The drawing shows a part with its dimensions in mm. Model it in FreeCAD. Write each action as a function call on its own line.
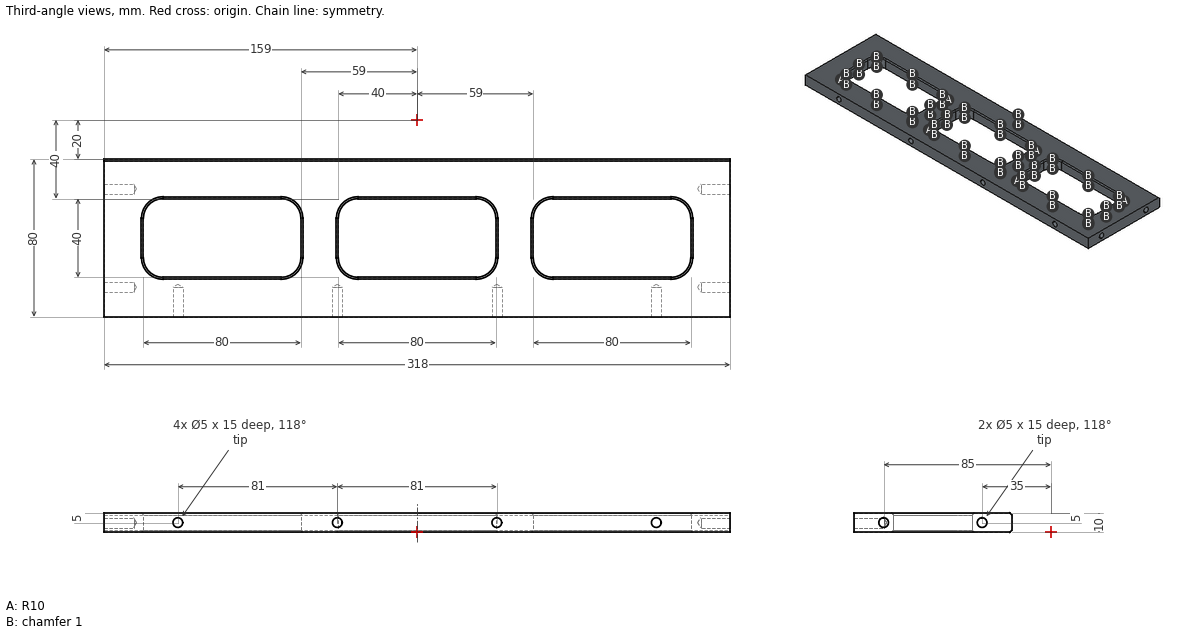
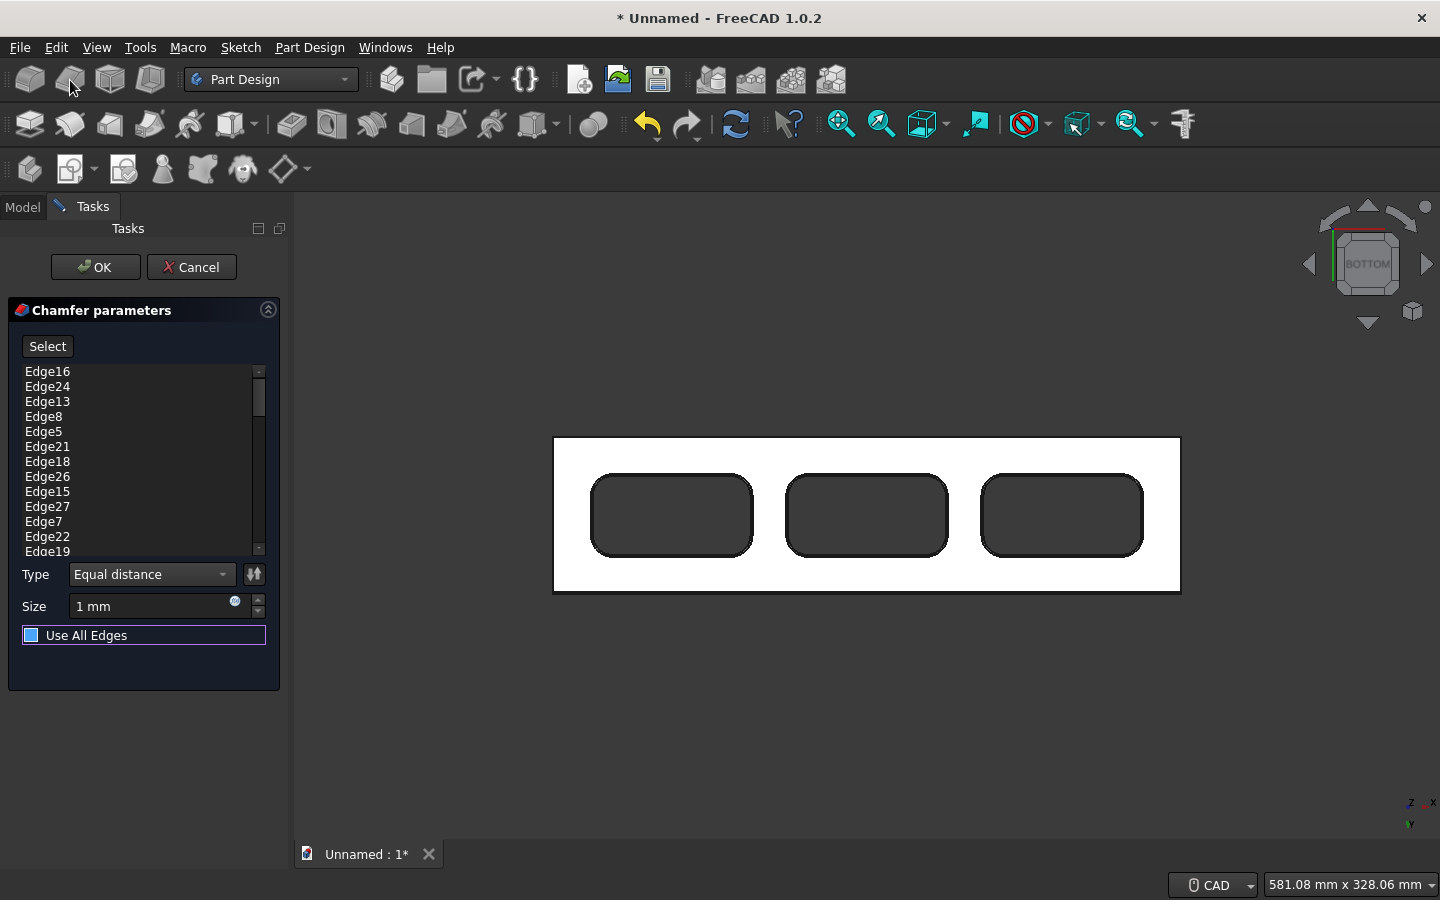
click(96, 267)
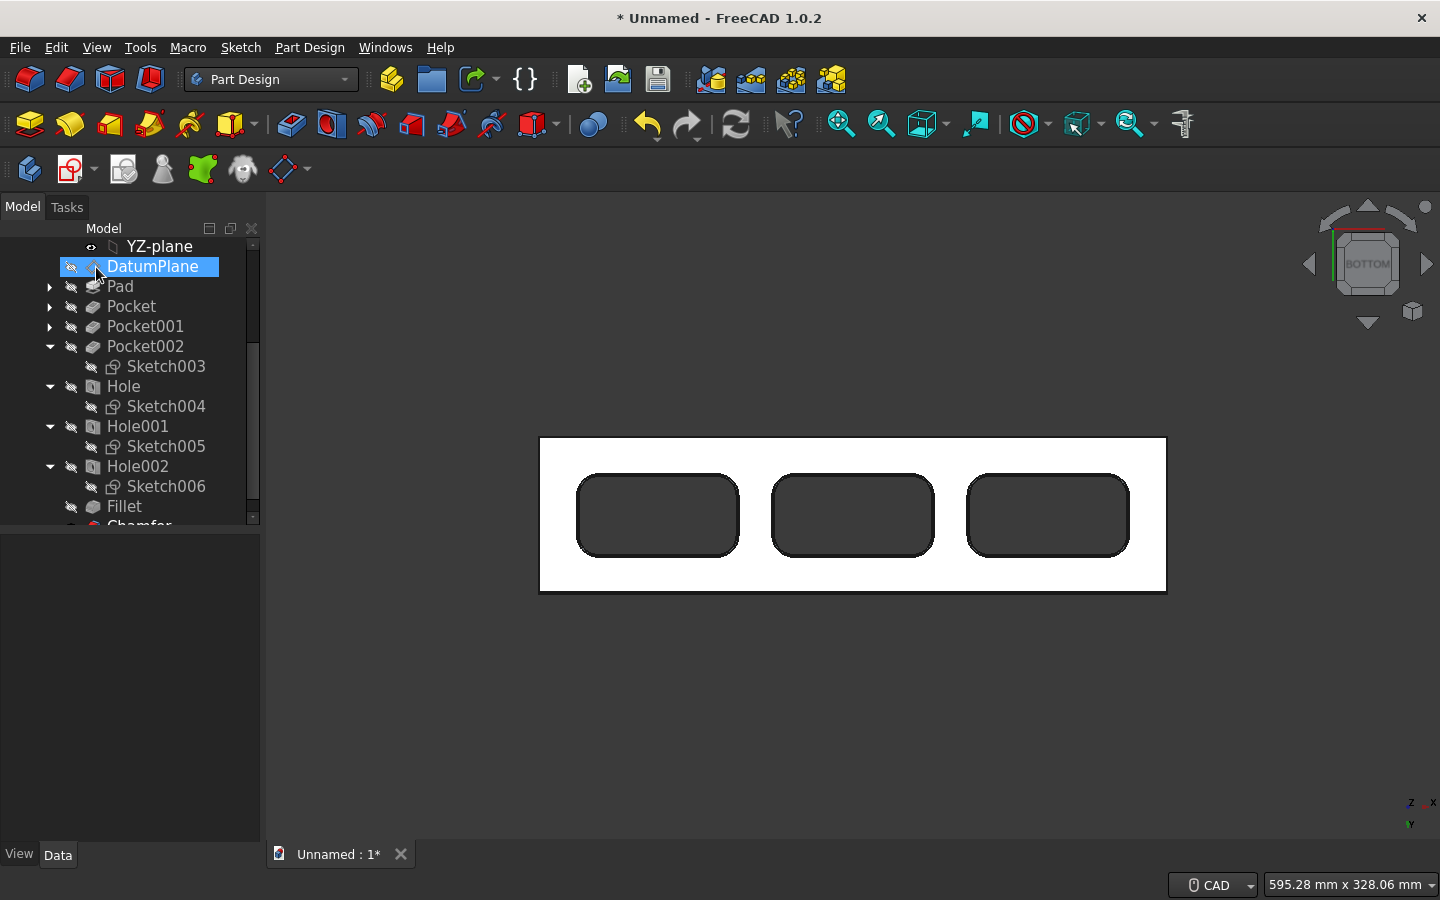
key(0)